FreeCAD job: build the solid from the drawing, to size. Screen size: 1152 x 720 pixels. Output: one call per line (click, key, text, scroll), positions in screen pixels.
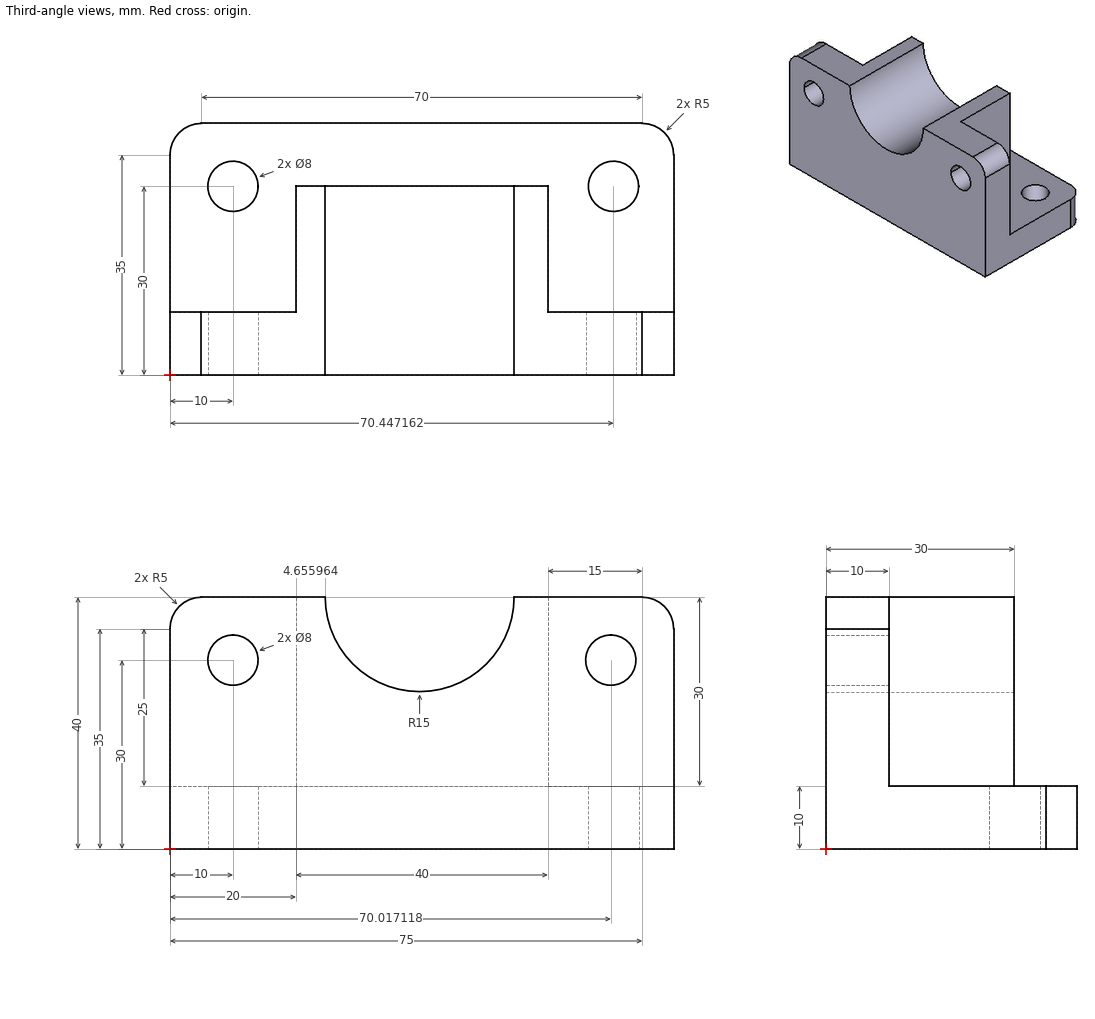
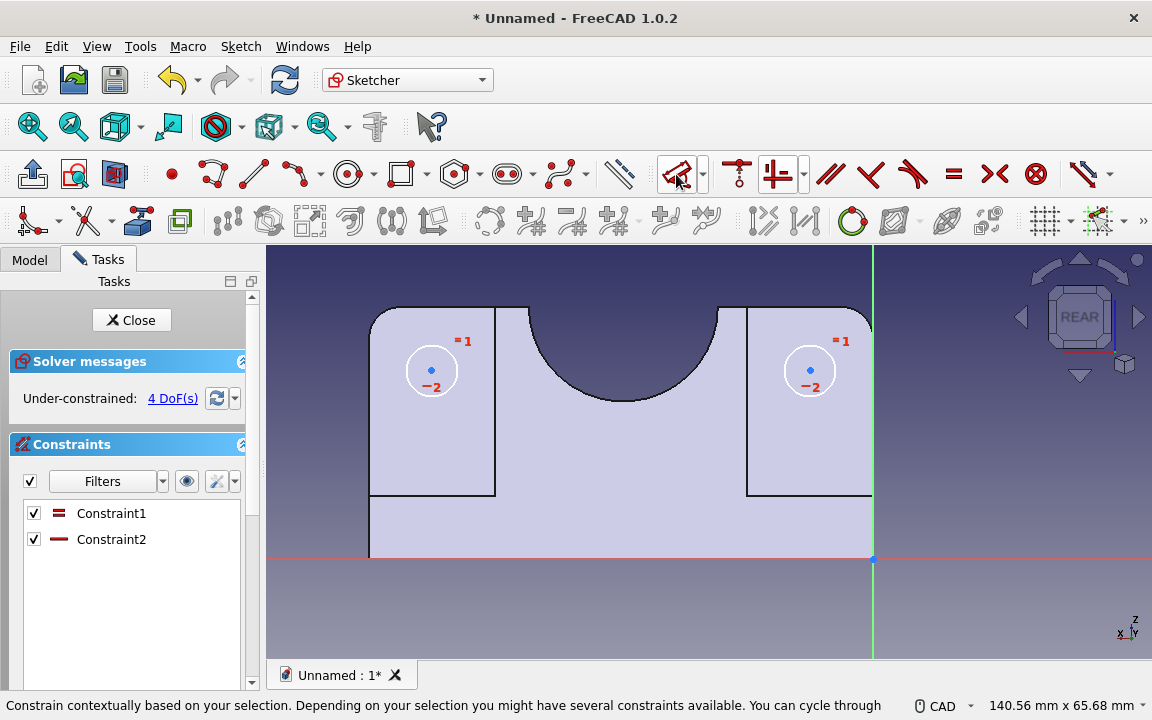
click(828, 353)
click(851, 330)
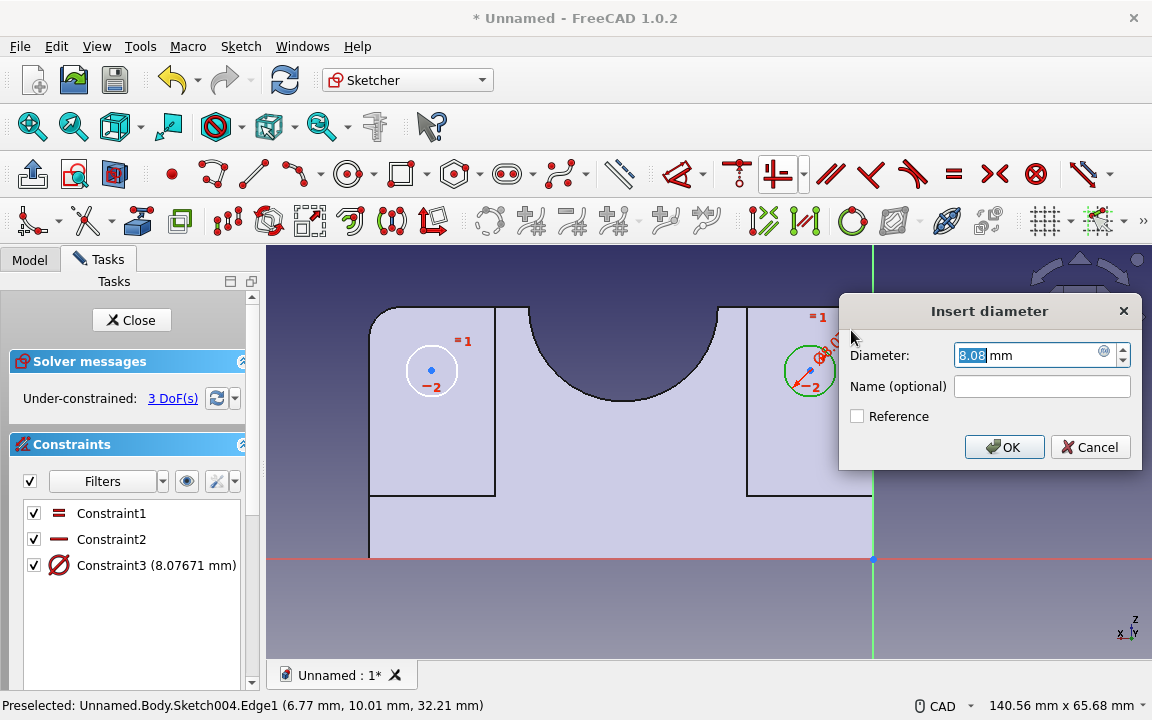
text(8)
key(Return)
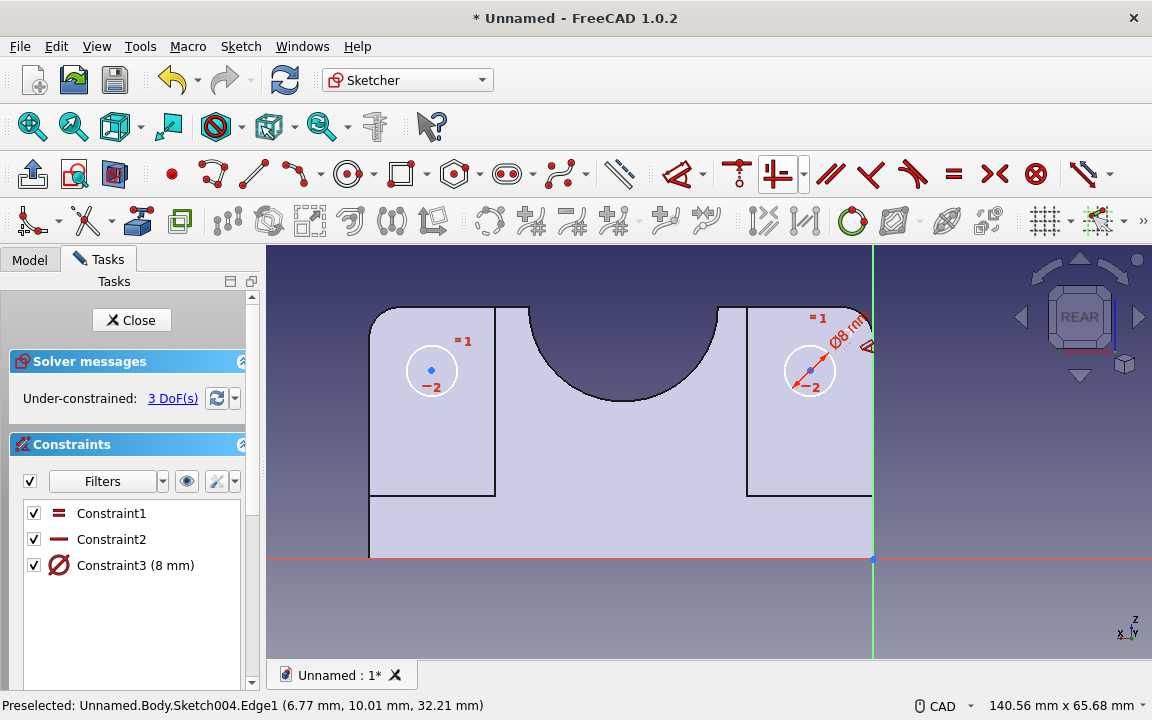
click(810, 371)
click(842, 593)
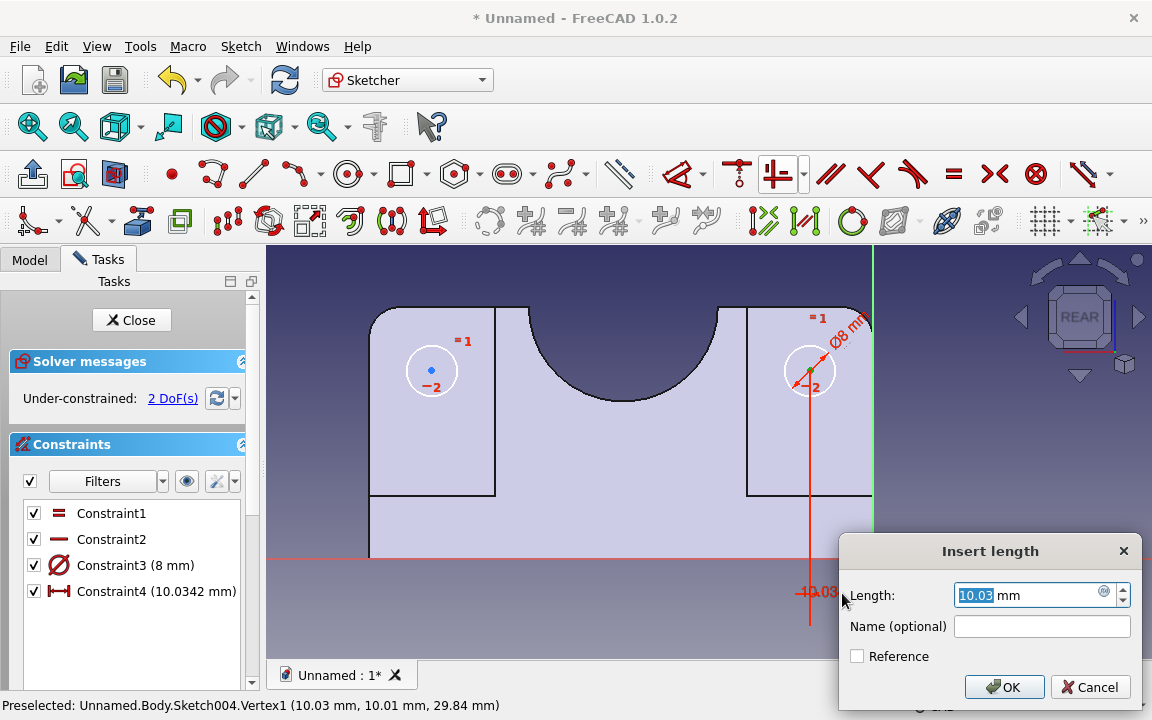
text(10)
key(Return)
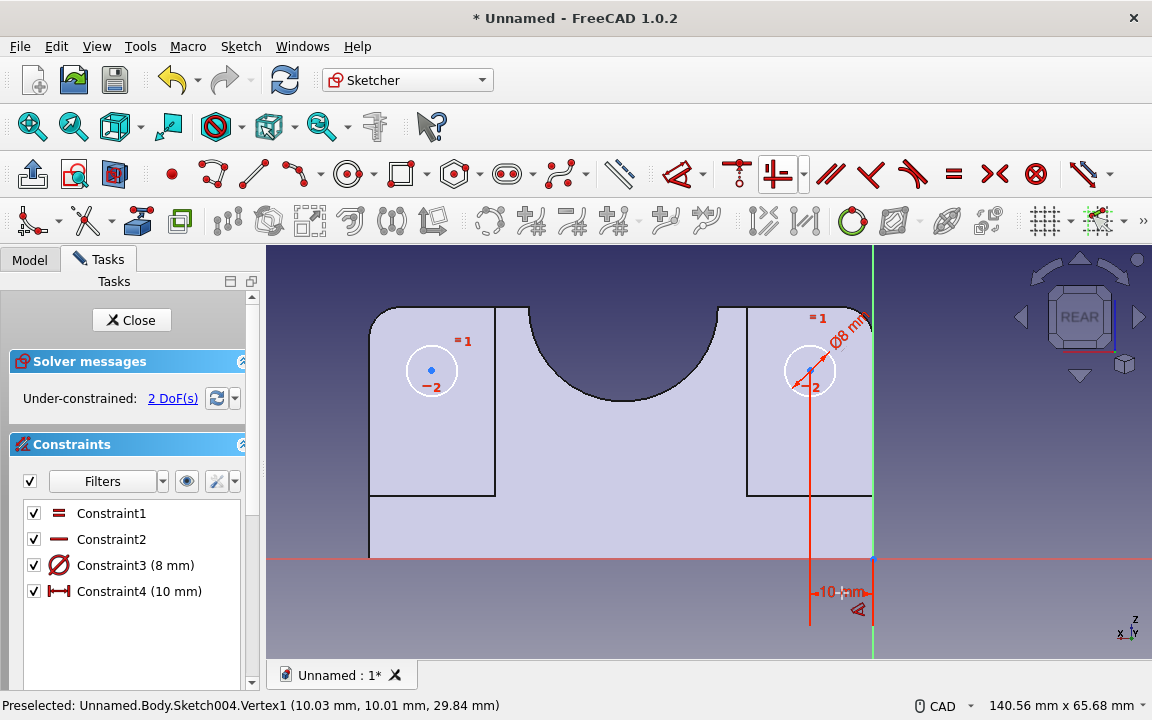
click(810, 371)
click(907, 465)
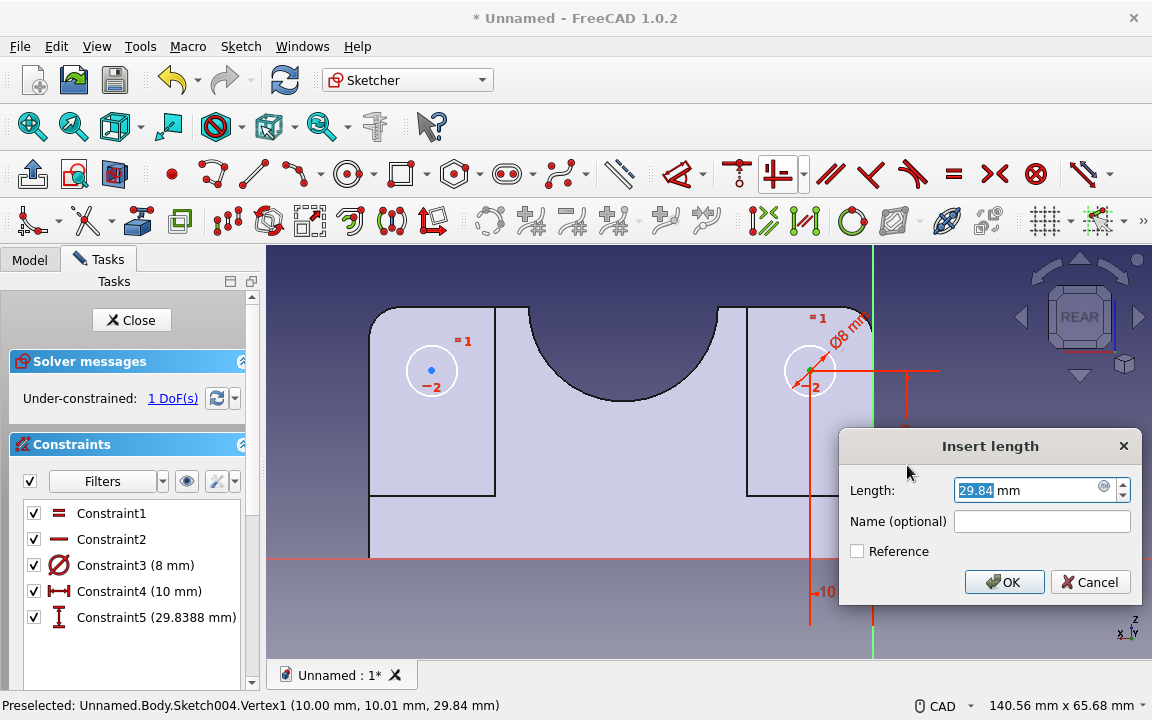
text(30)
key(Return)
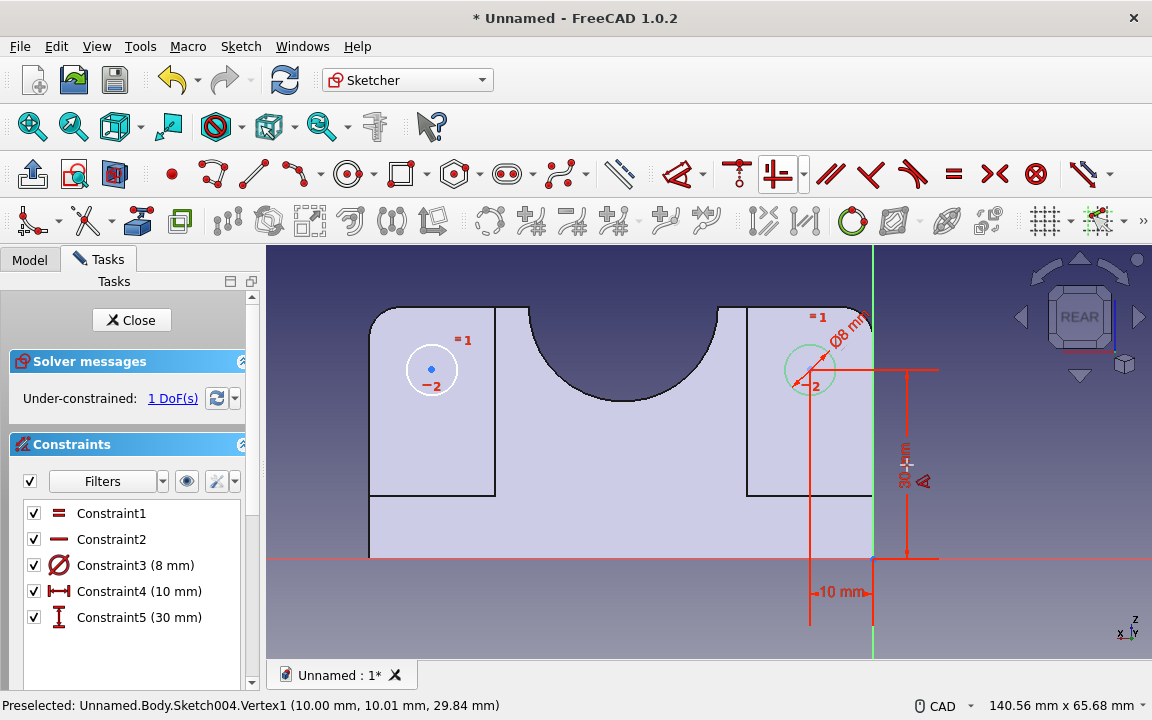
click(432, 370)
click(653, 593)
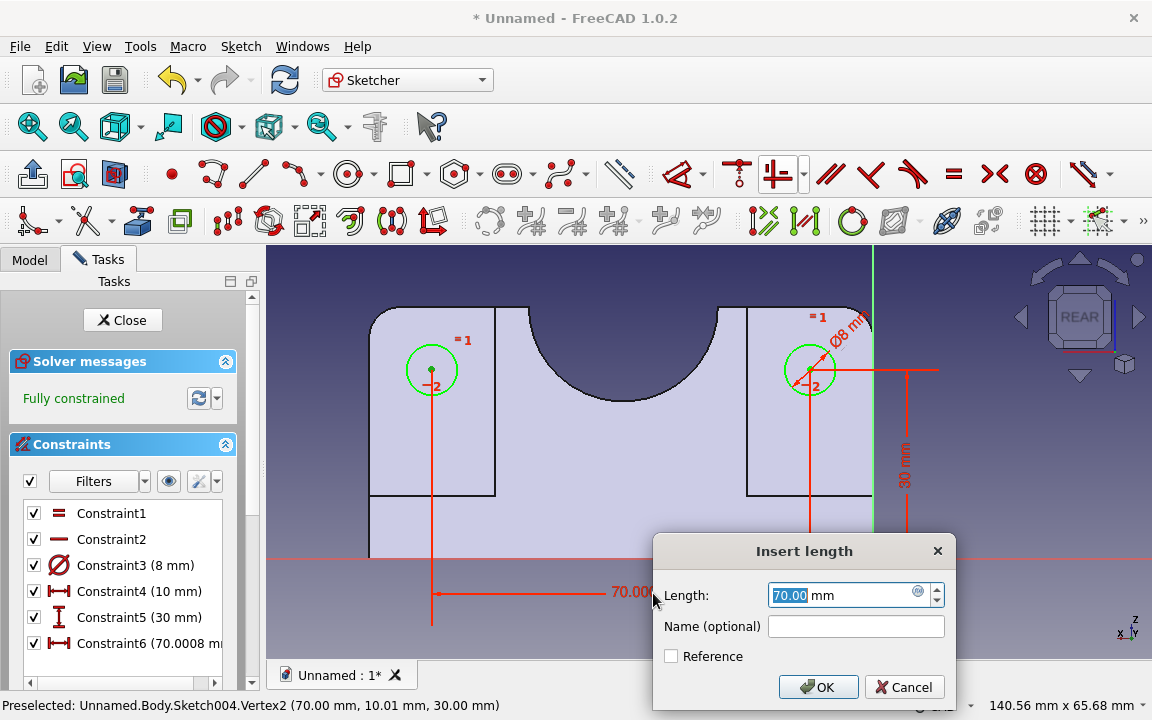
text(70.017118)
key(Return)
key(Escape)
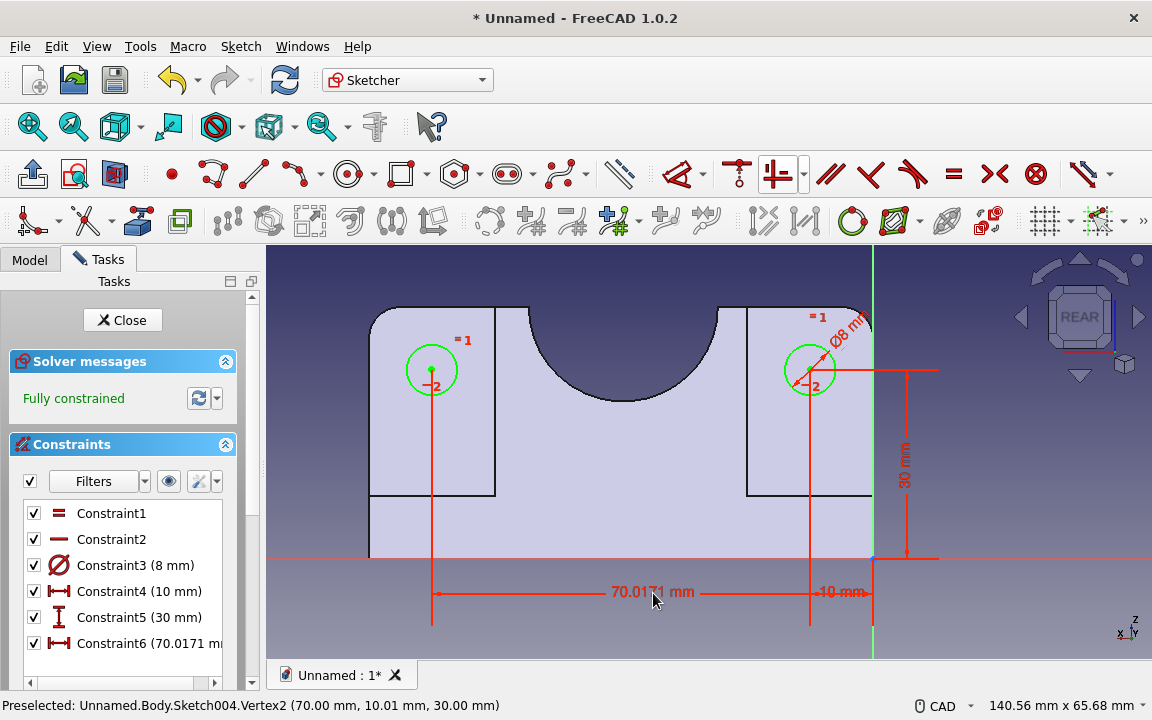
click(123, 320)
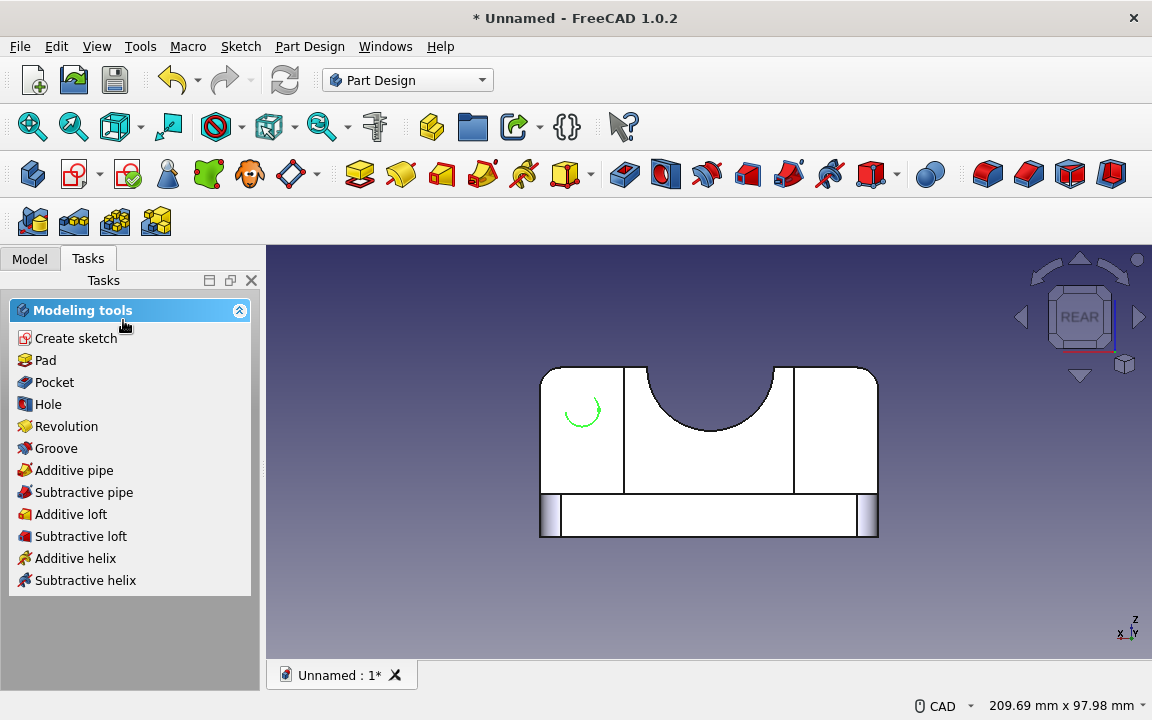
click(625, 174)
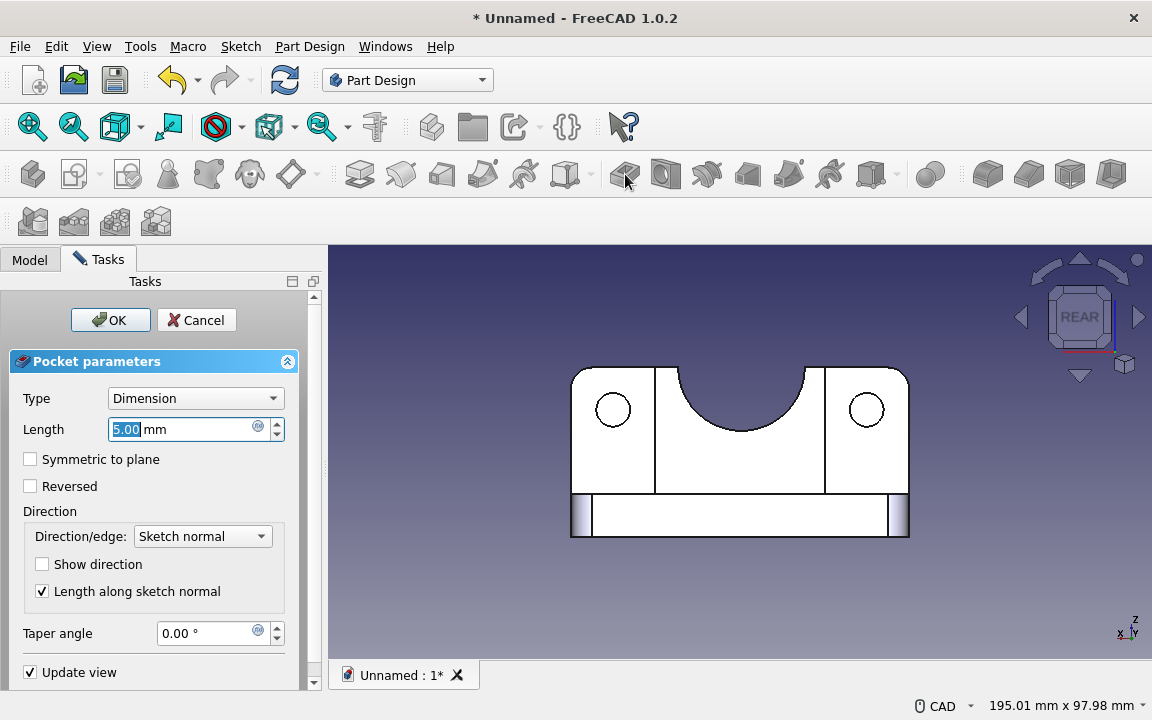
text(10)
key(Tab)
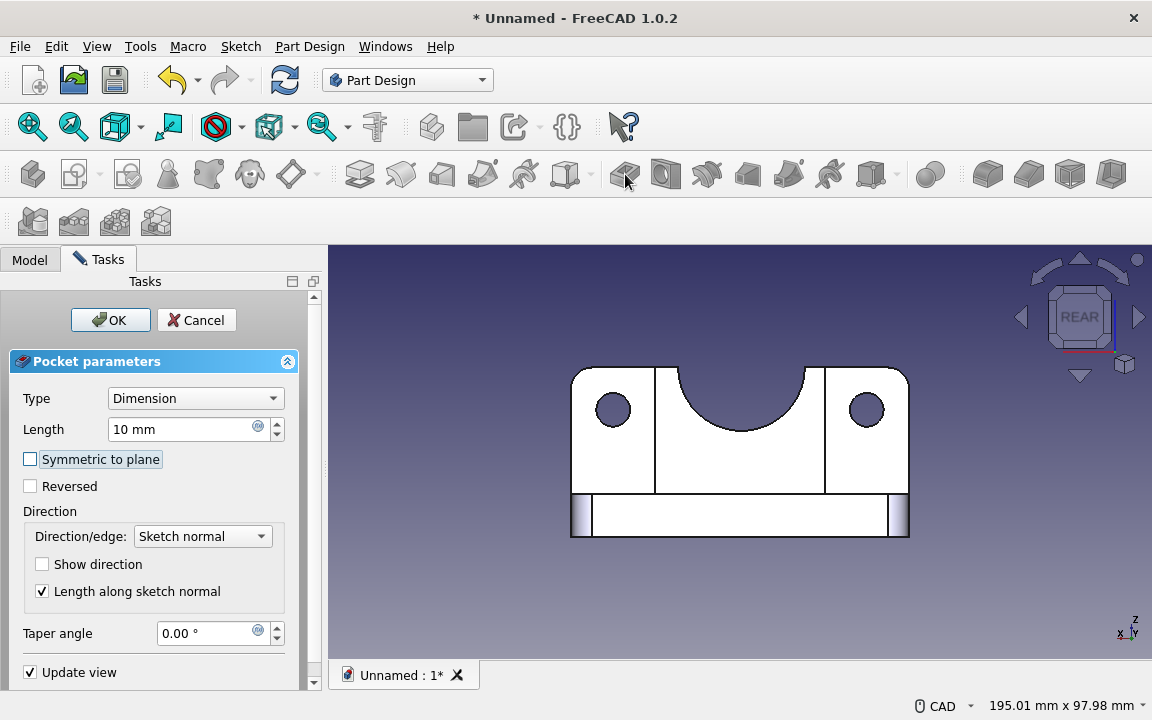
click(111, 320)